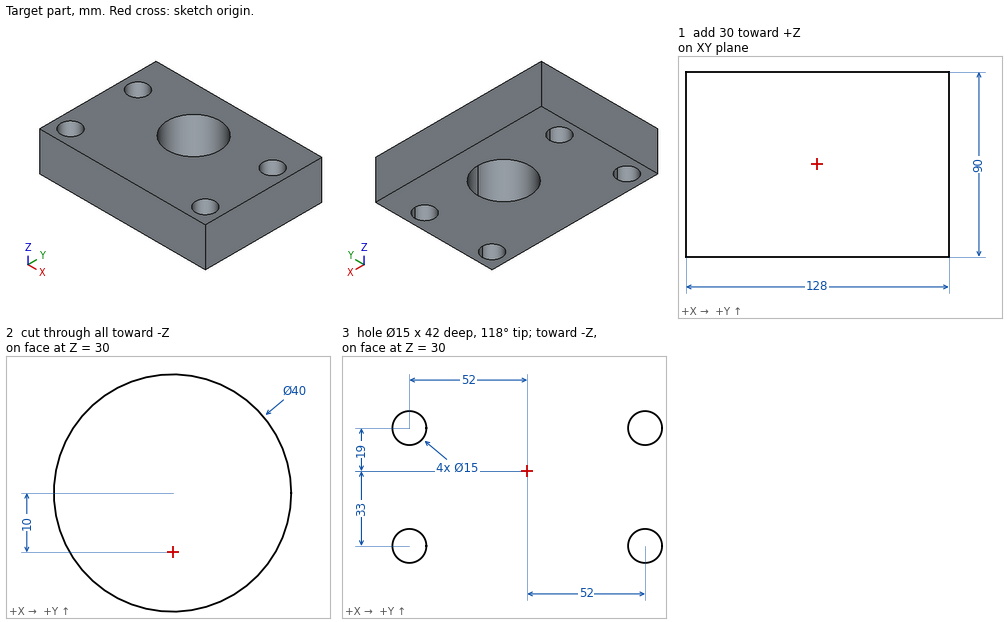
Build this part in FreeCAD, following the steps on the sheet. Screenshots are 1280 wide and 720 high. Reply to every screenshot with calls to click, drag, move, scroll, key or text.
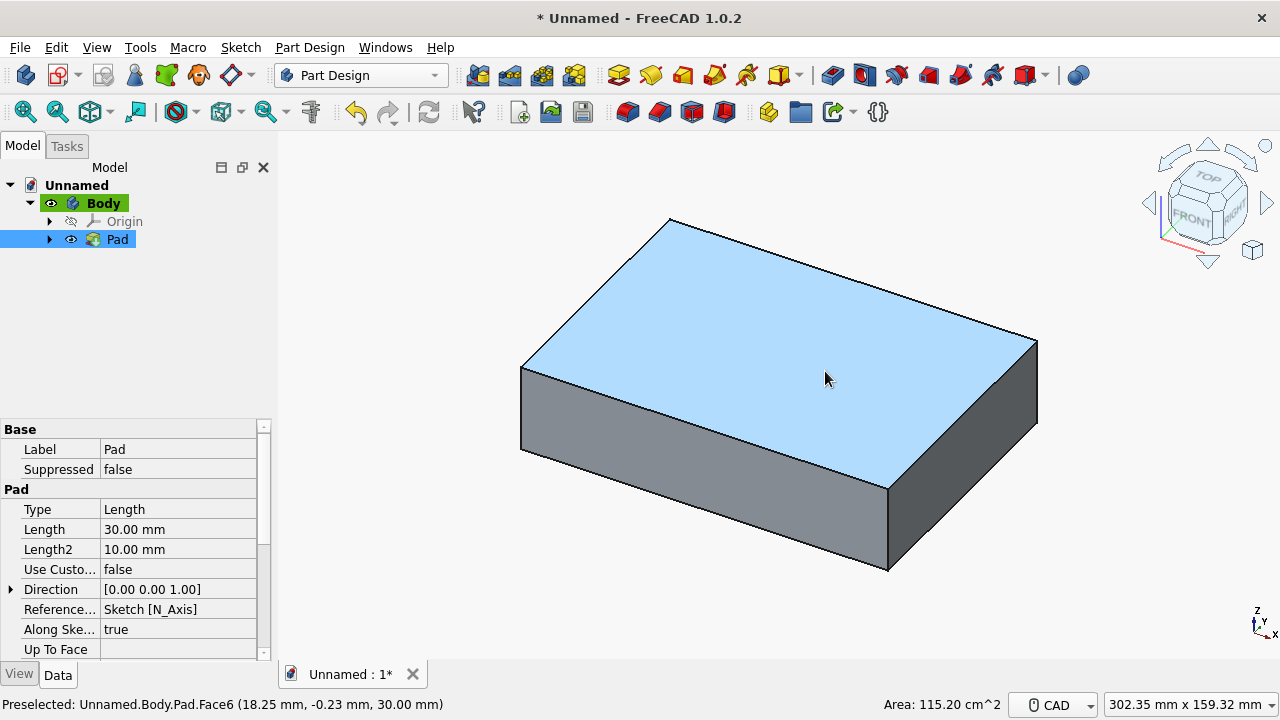
click(58, 76)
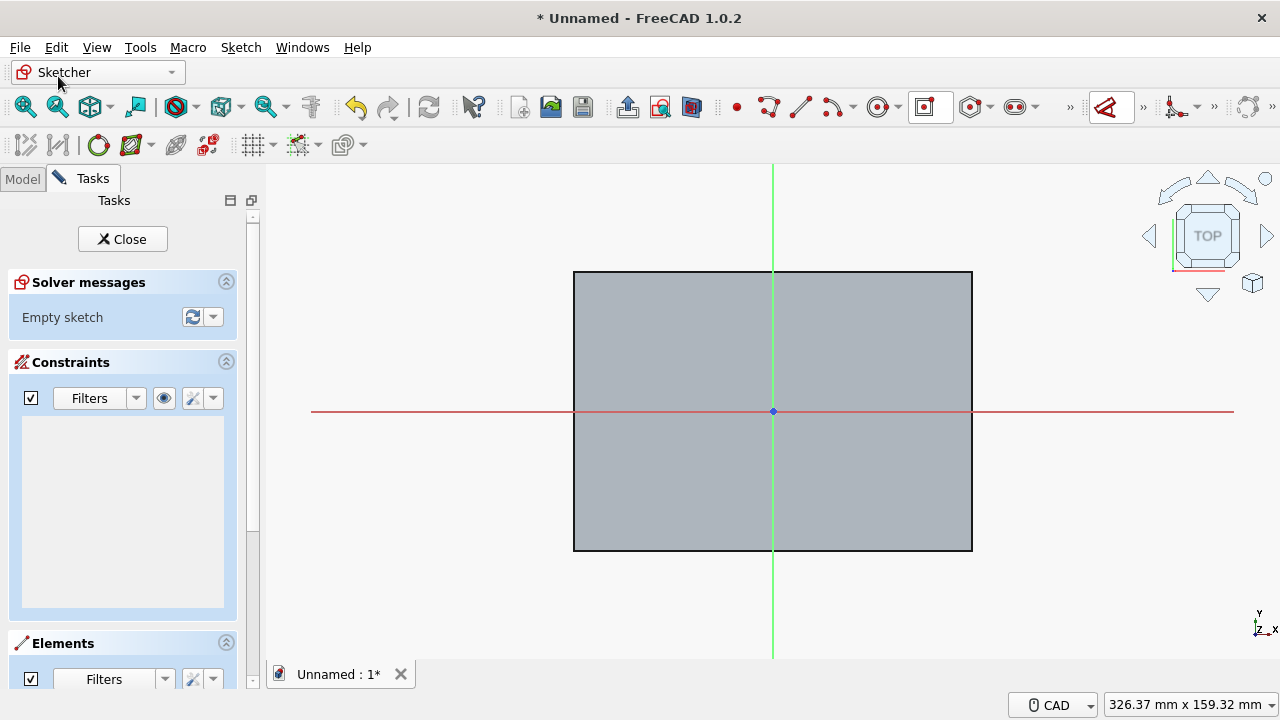
scroll(813, 362, up, 5)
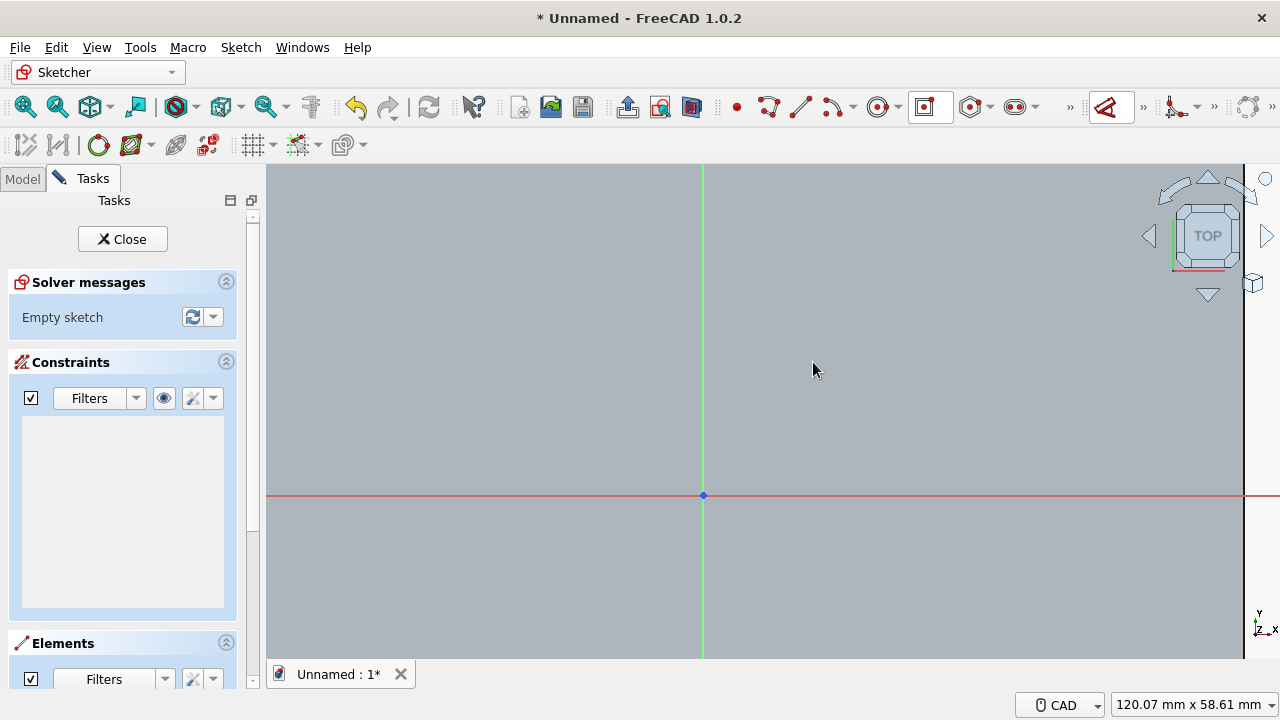
click(878, 108)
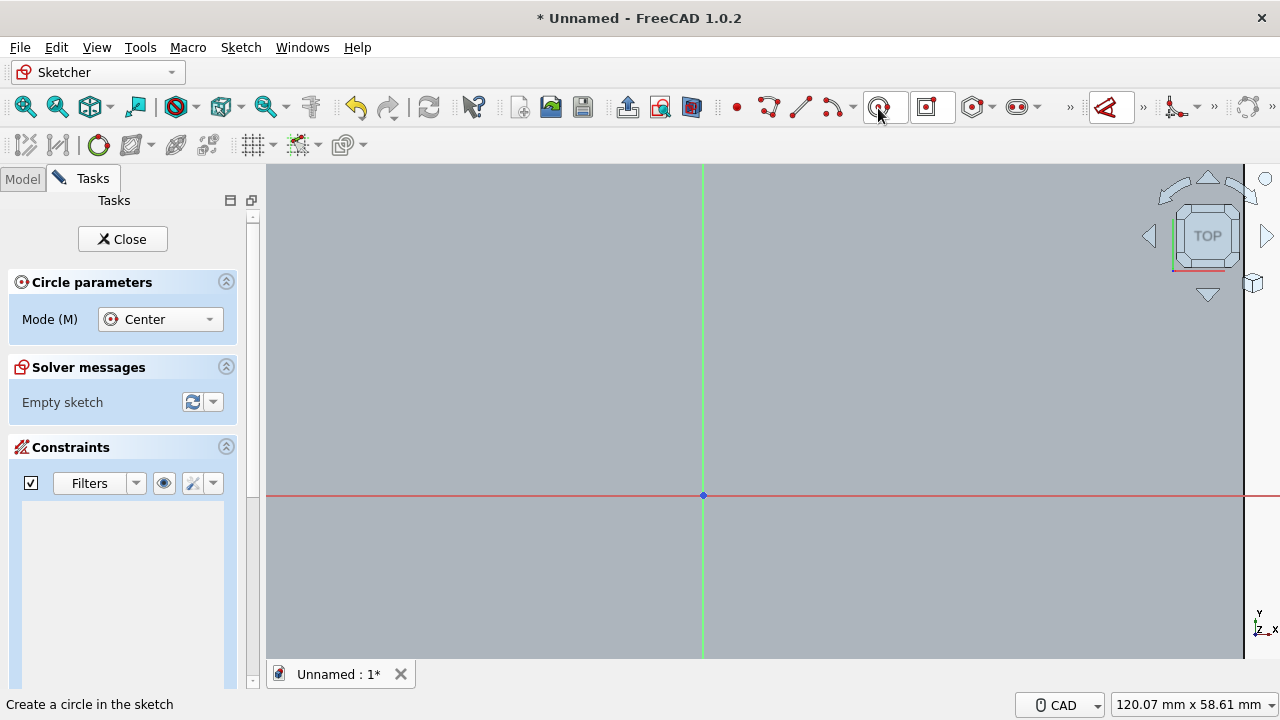
click(703, 411)
click(823, 292)
key(Escape)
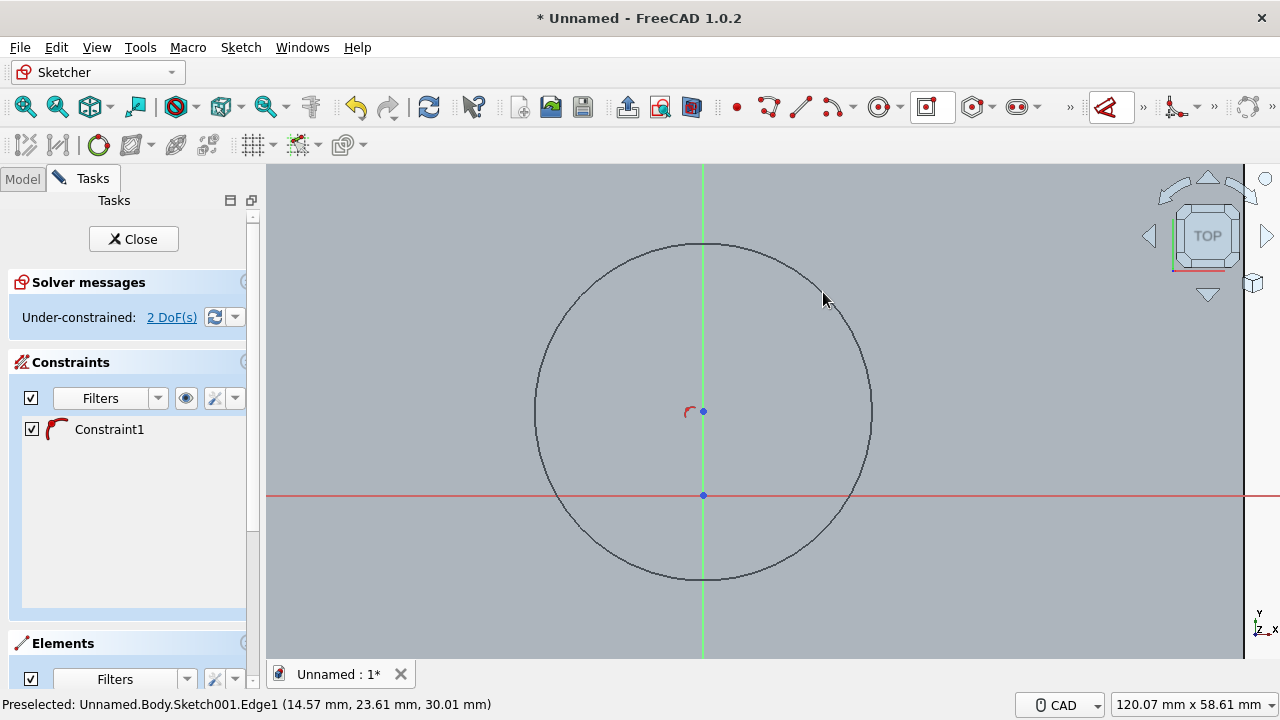
click(822, 292)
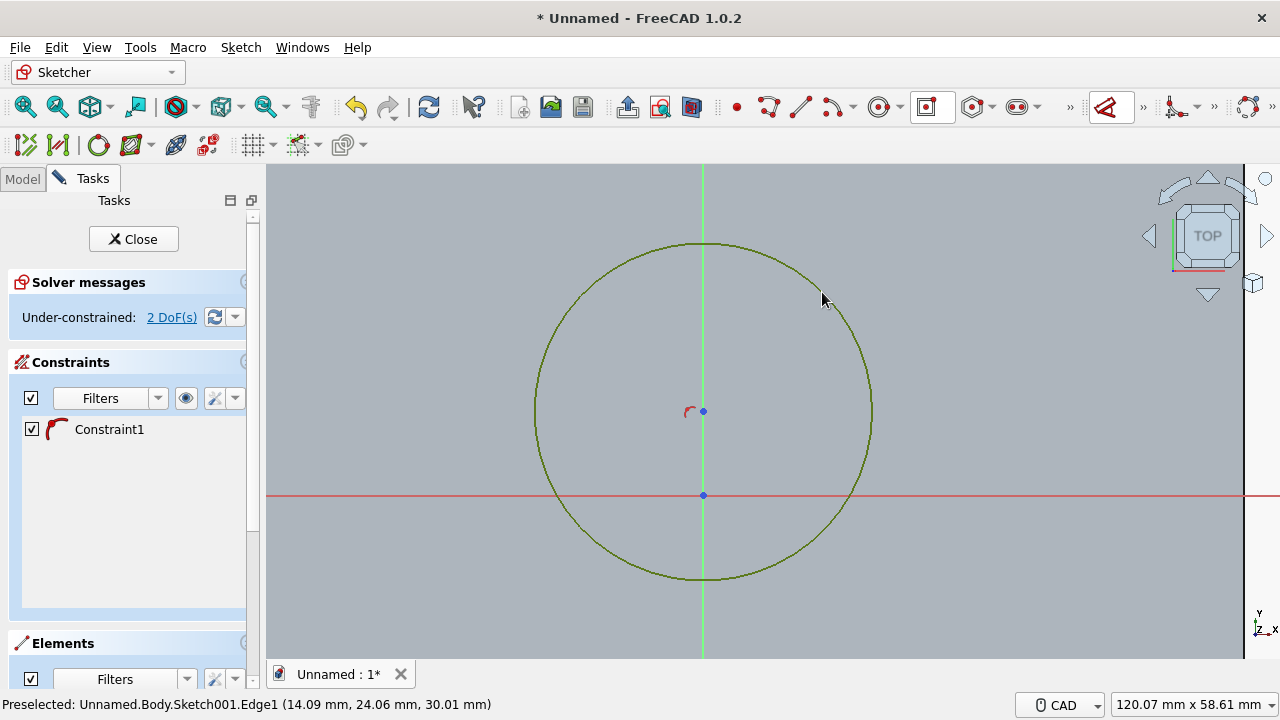
click(1128, 108)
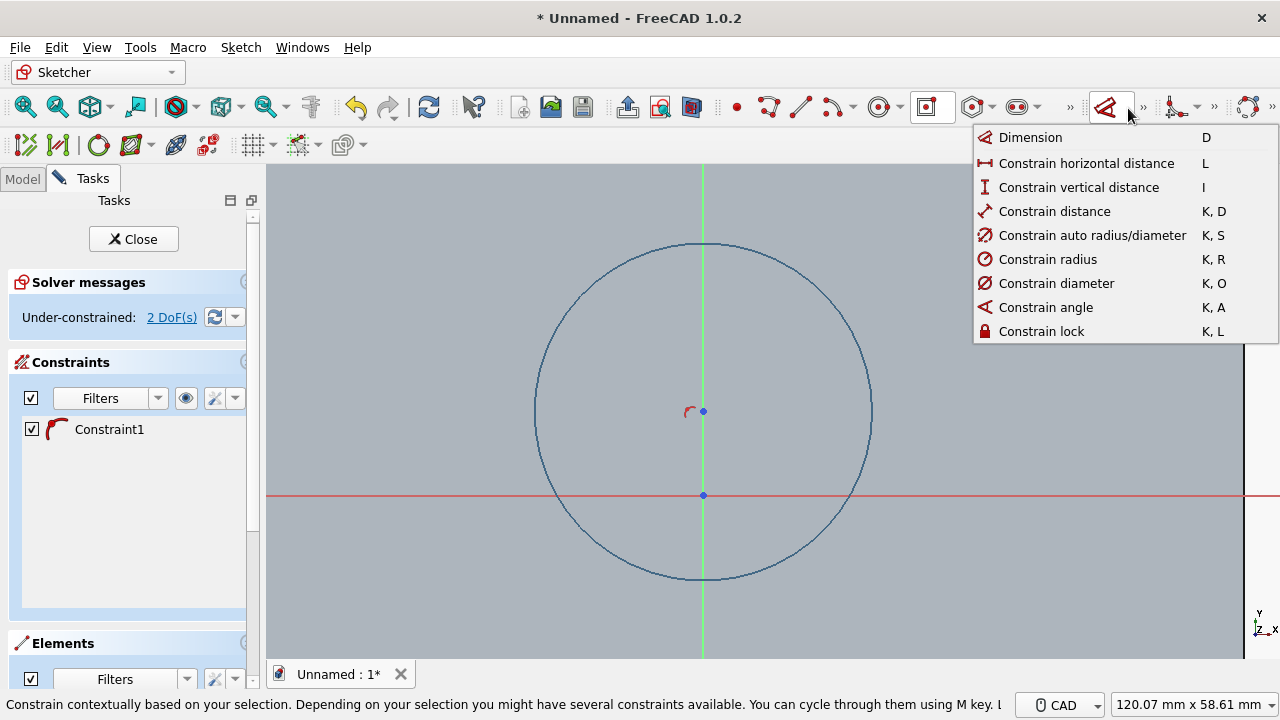
click(1126, 283)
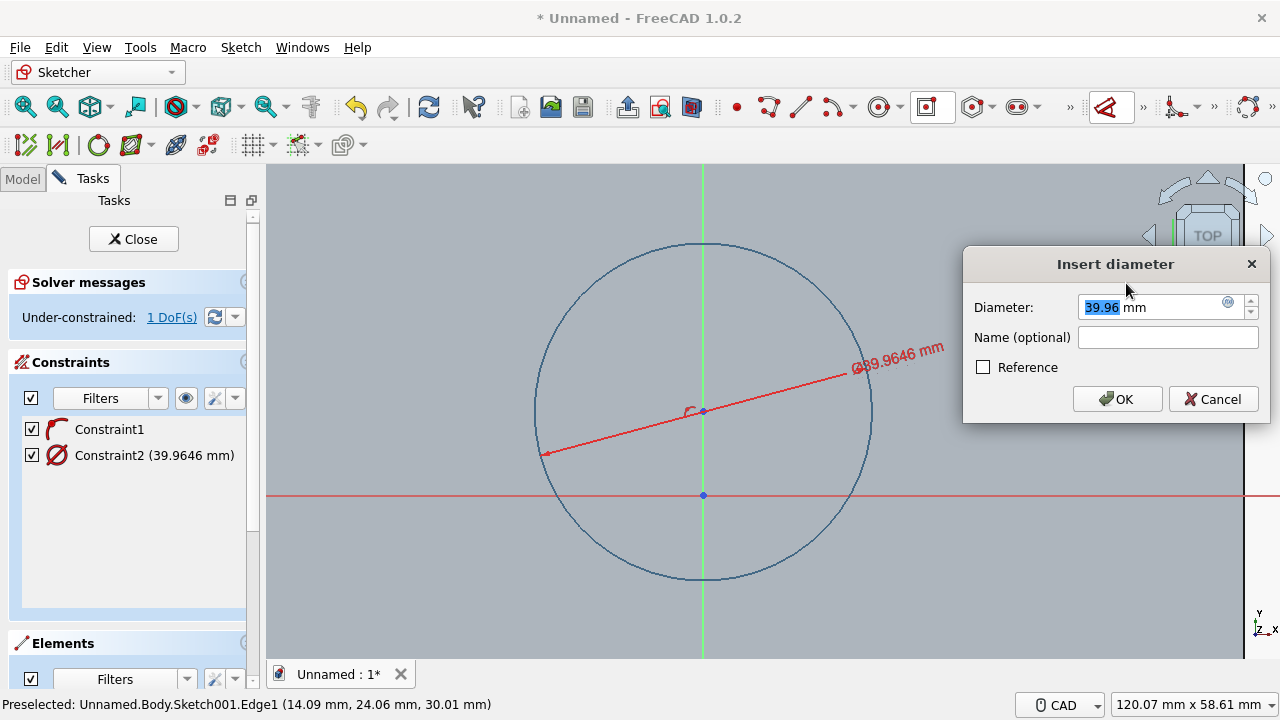
text(40)
key(Return)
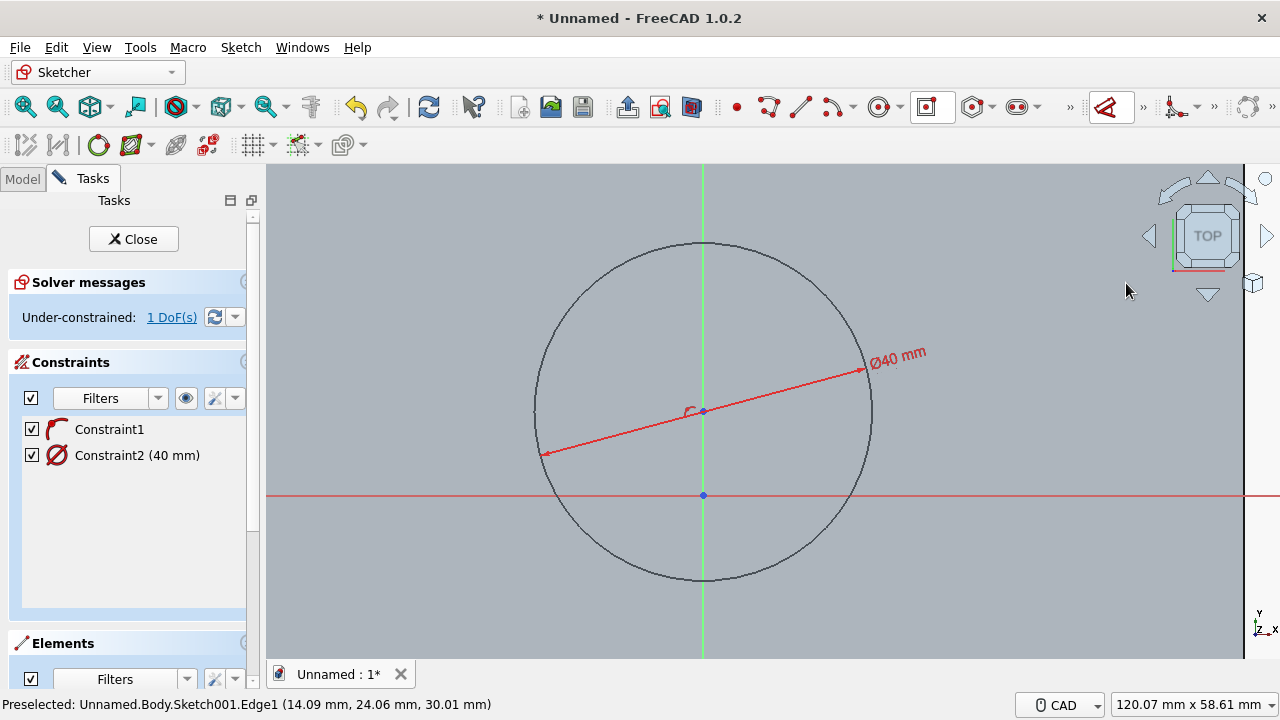
click(703, 412)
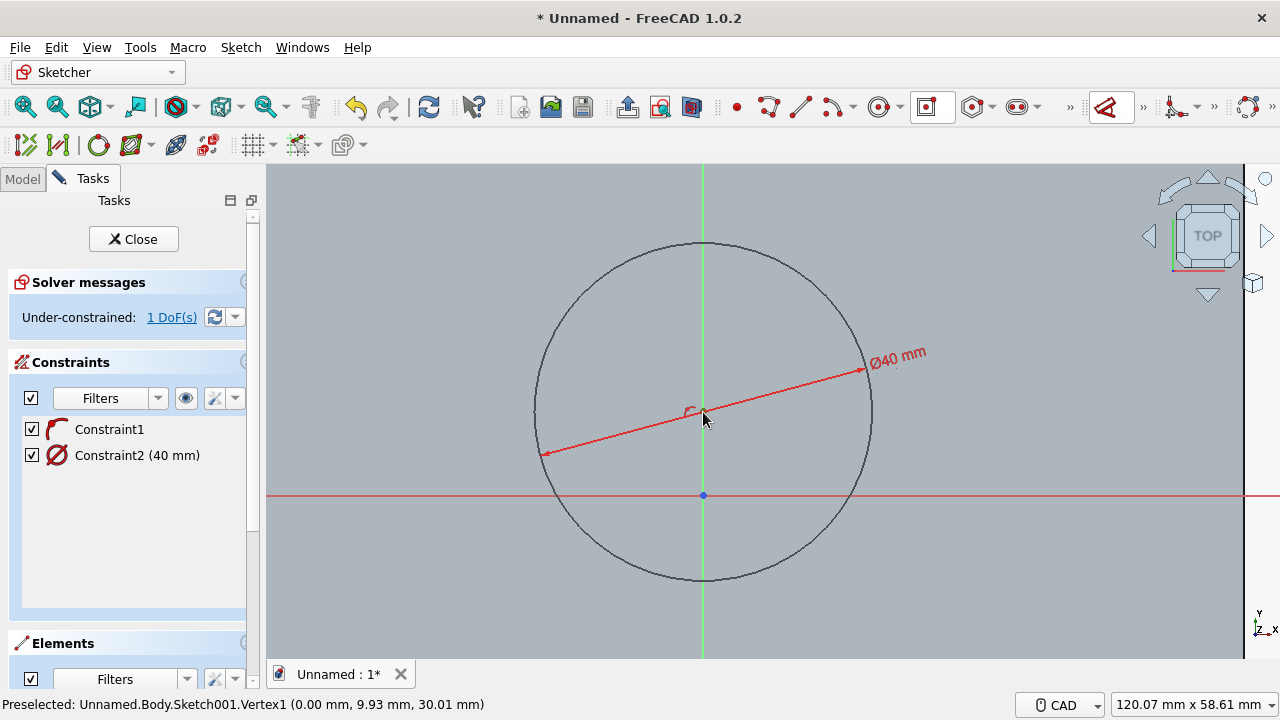
key(i)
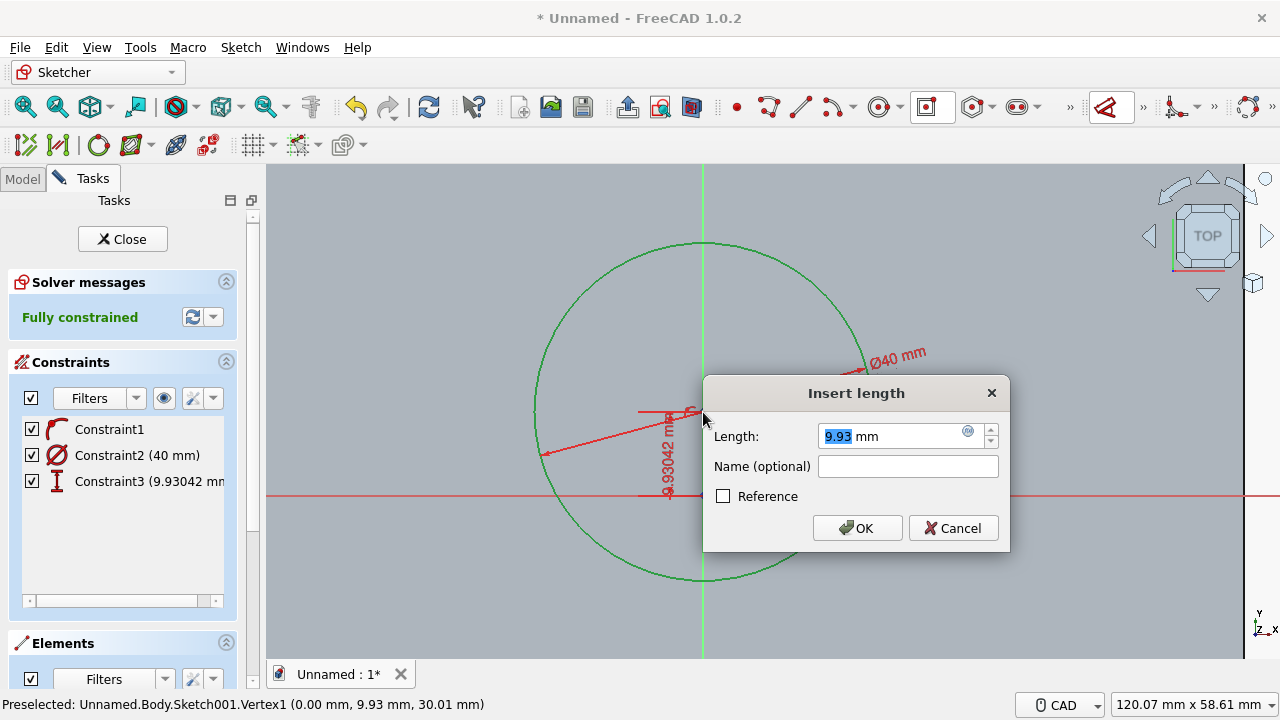
text(10)
key(Return)